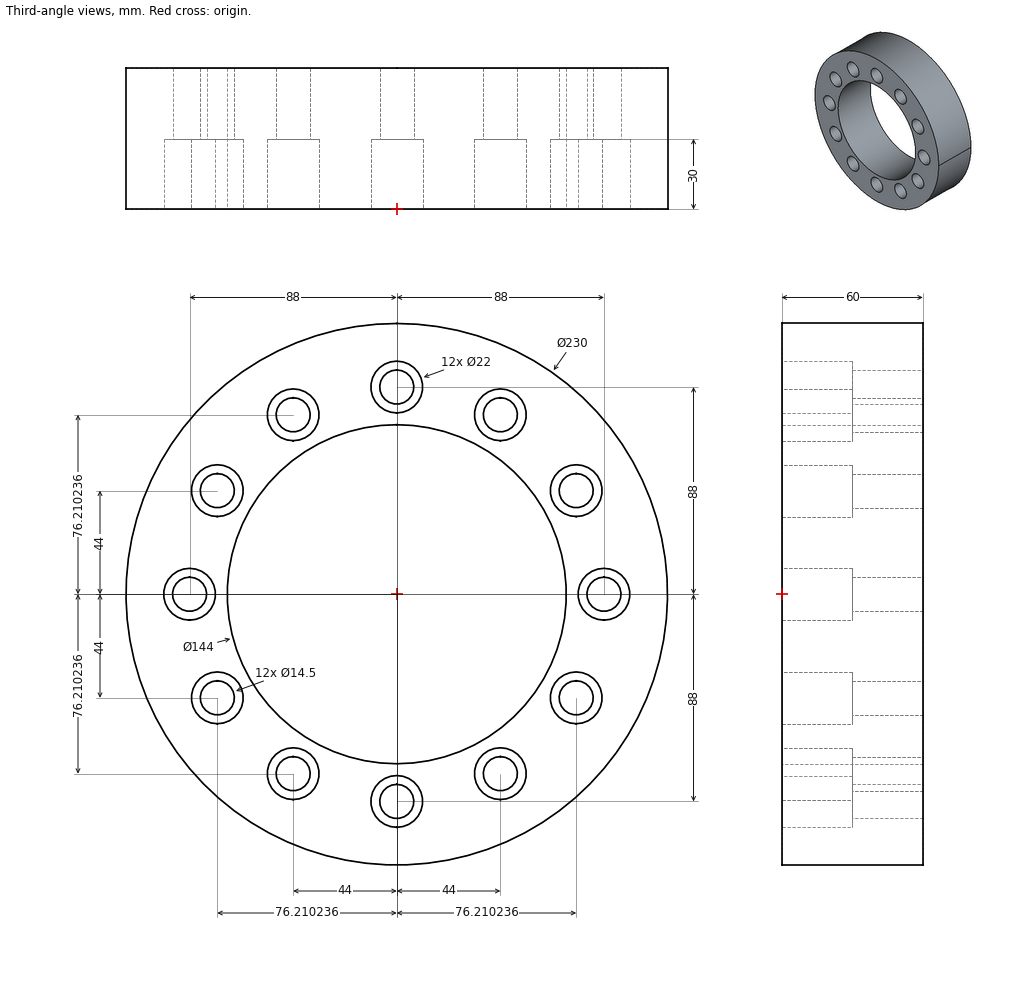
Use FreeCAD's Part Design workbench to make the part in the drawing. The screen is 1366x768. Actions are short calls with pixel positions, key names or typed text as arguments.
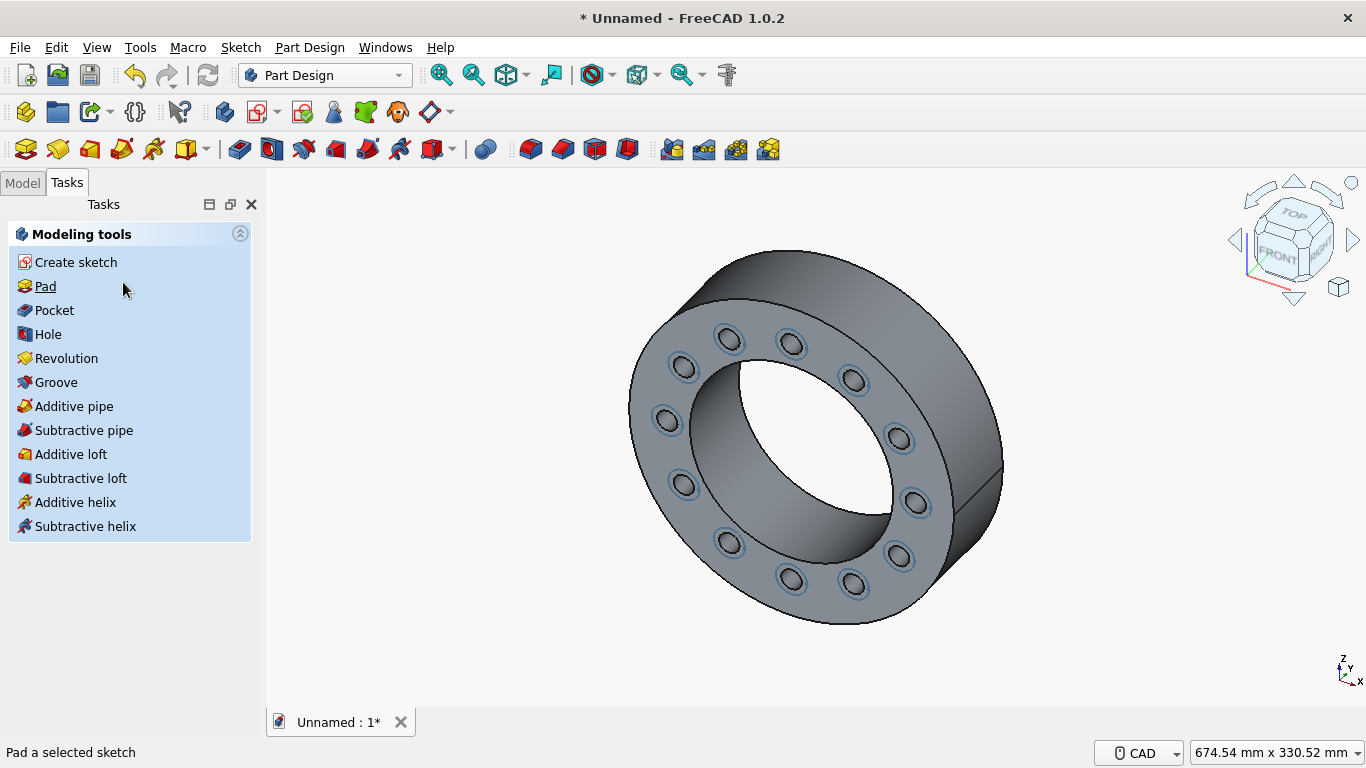
click(240, 150)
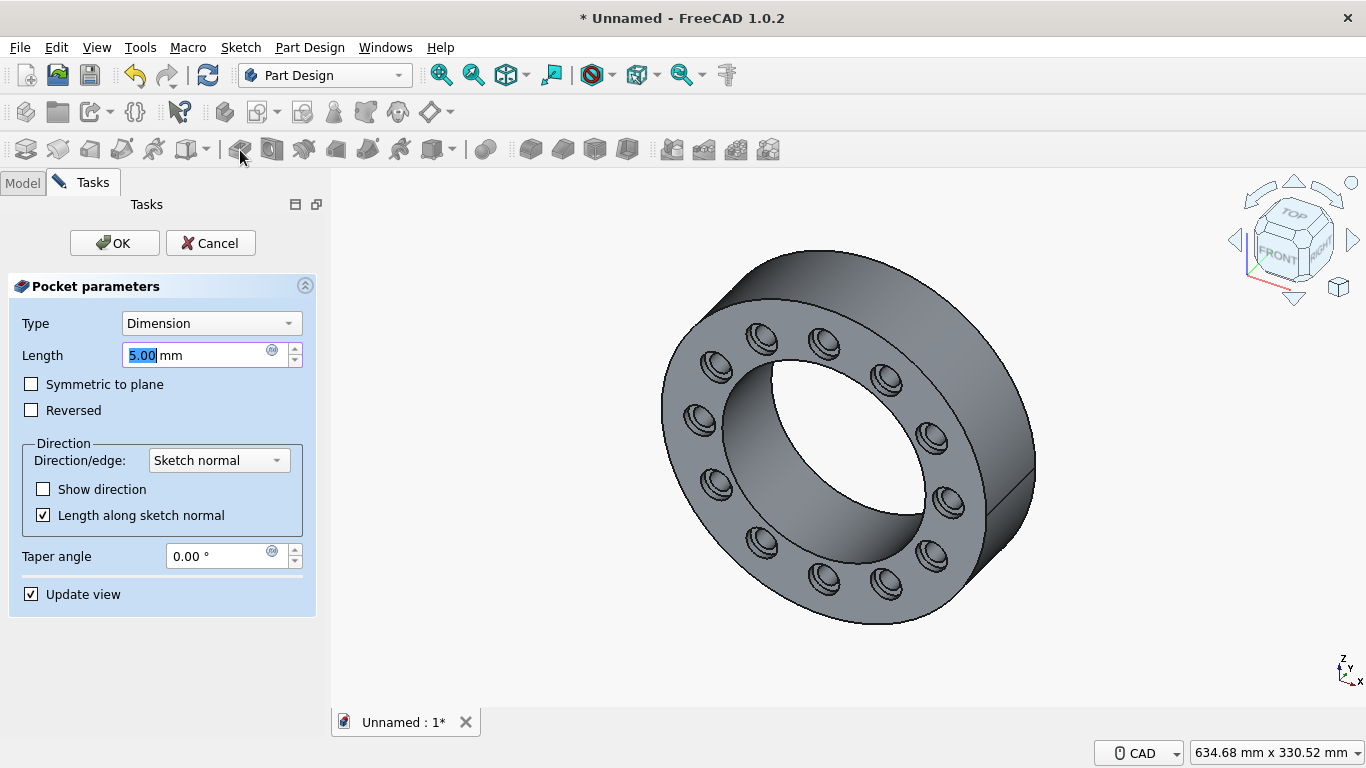
text(30)
key(Tab)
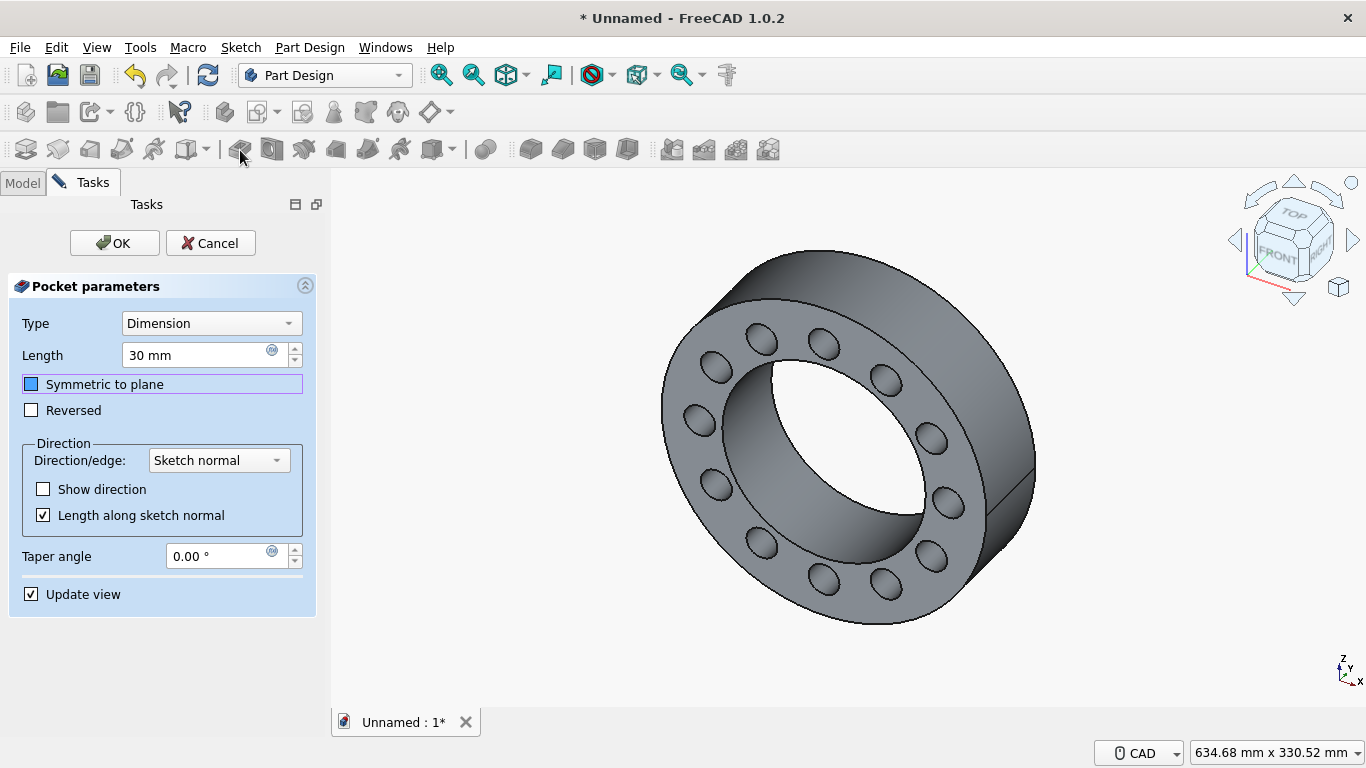
click(115, 243)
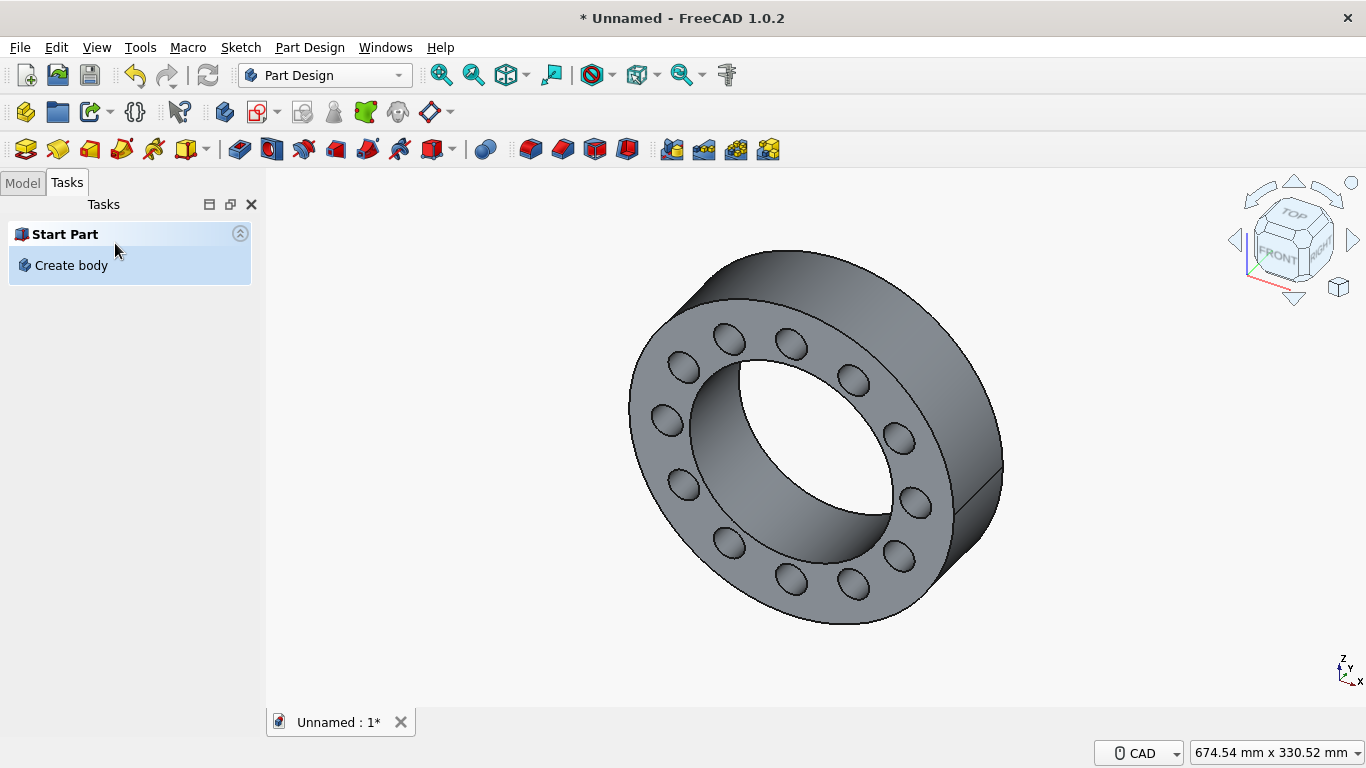
key(0)